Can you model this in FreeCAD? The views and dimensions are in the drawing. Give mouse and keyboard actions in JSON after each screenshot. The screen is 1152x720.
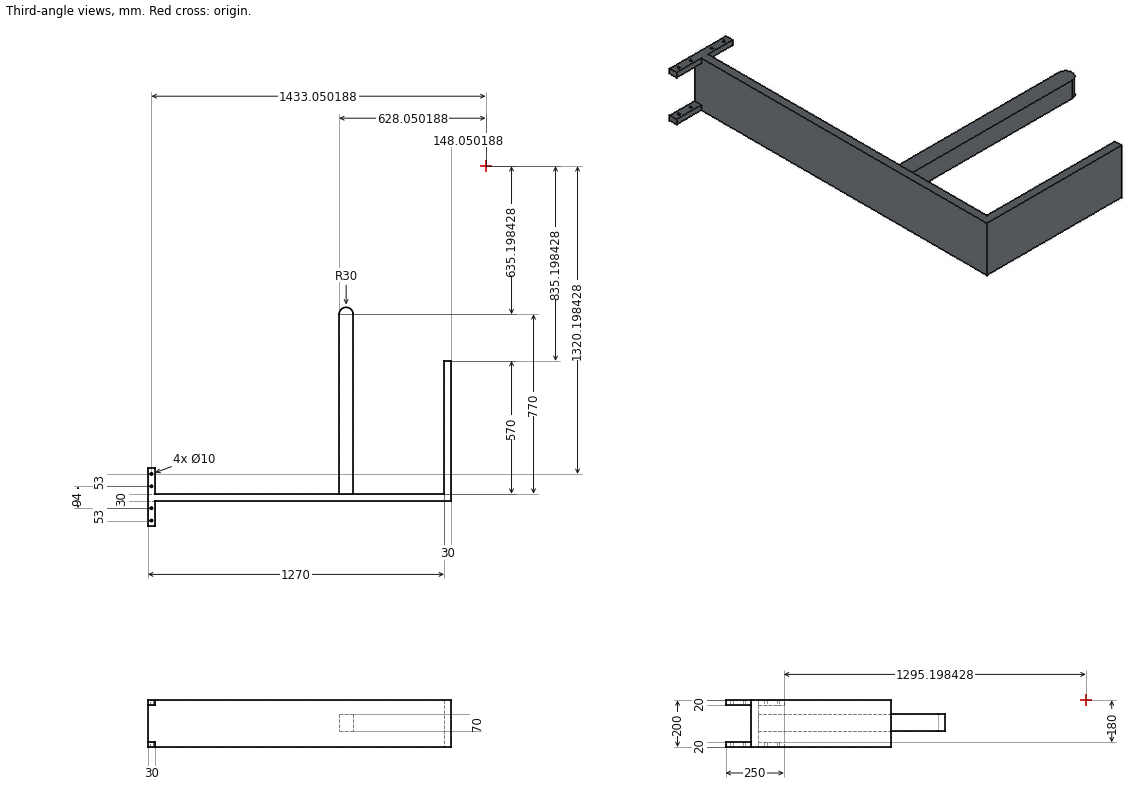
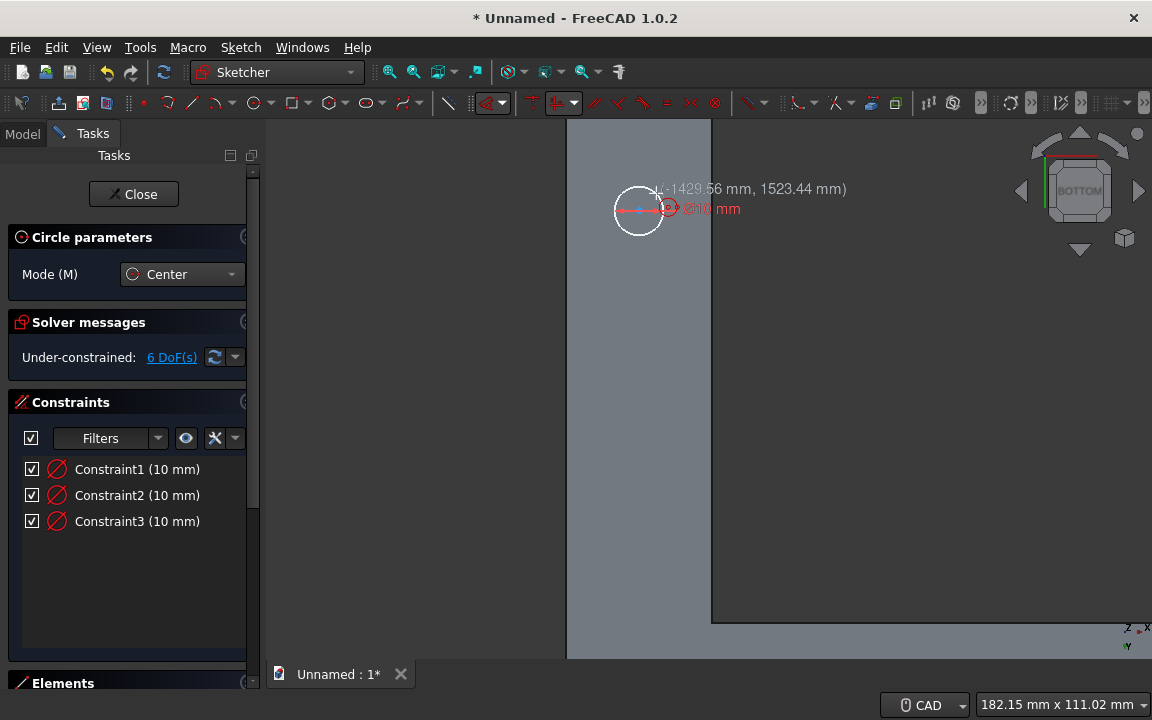
{"action": "left_click", "coordinate": [639, 468]}
{"action": "mouse_move", "coordinate": [656, 450]}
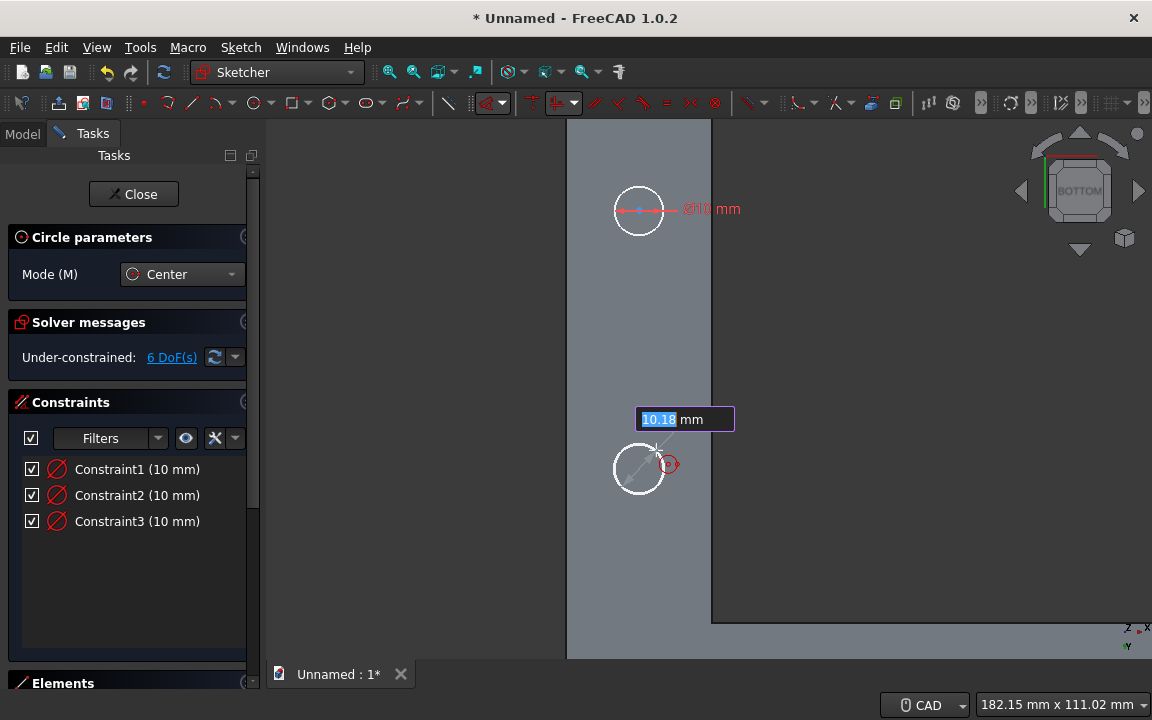
{"action": "type", "text": "10"}
{"action": "key", "text": "Return"}
{"action": "key", "text": "Escape"}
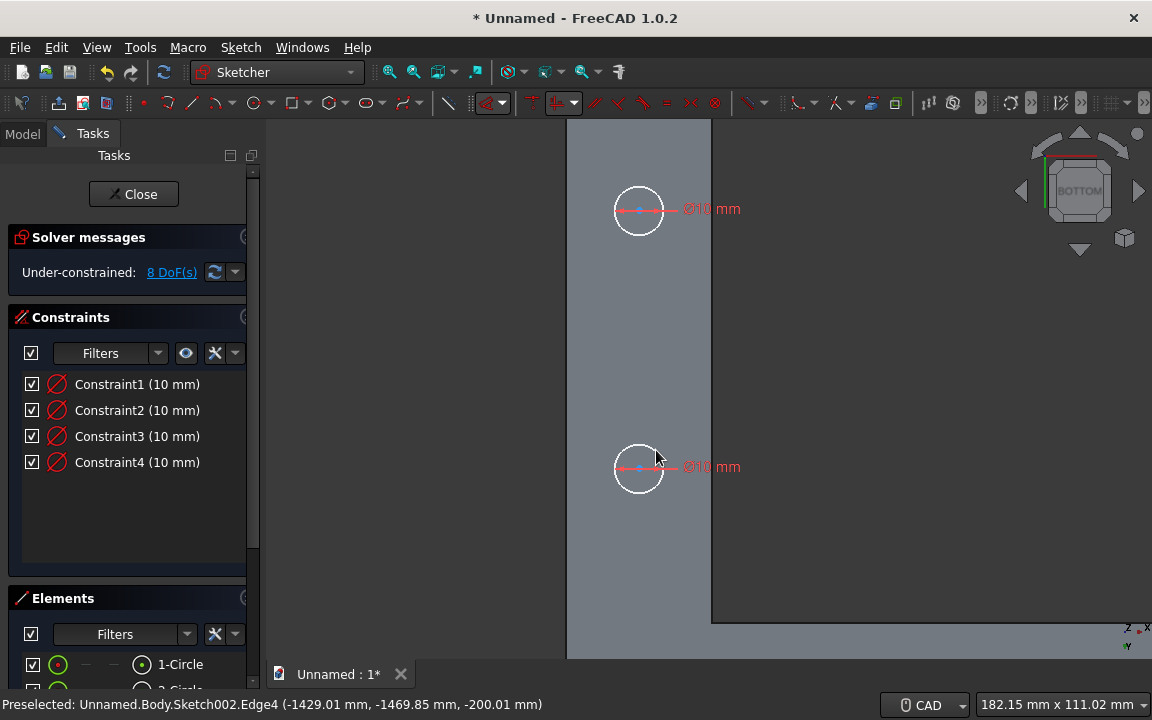
{"action": "scroll", "coordinate": [641, 210], "scroll_direction": "down", "scroll_amount": 5}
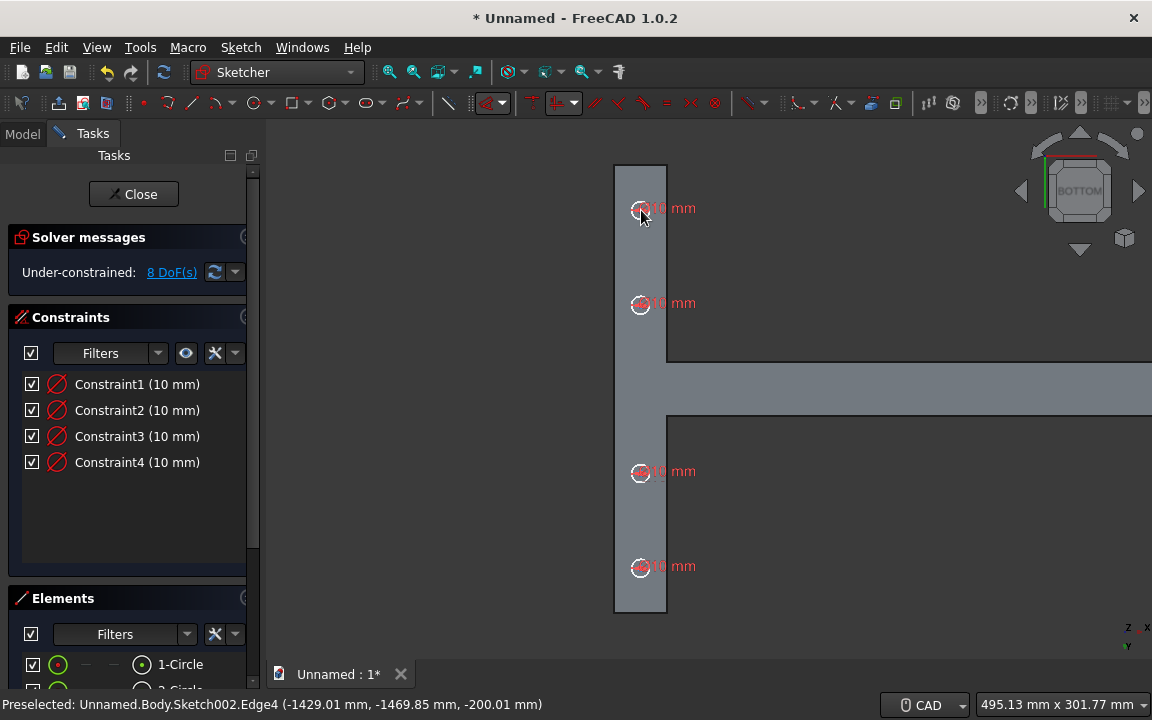
{"action": "left_click", "coordinate": [641, 568]}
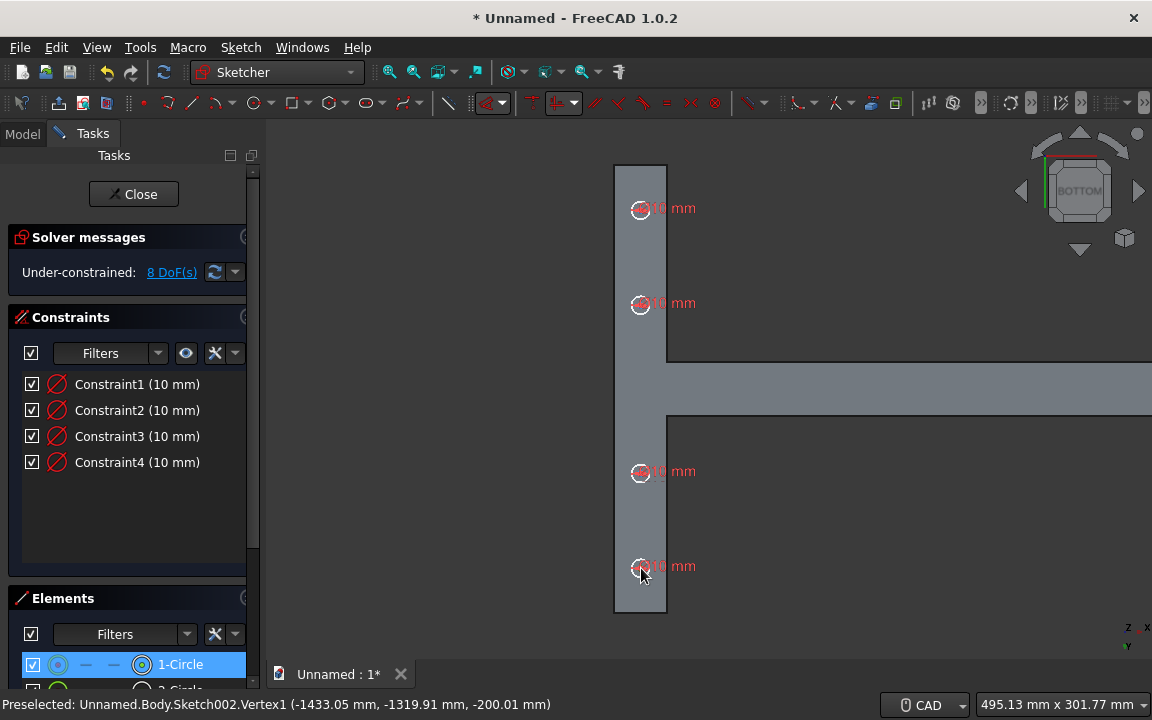
{"action": "left_click", "coordinate": [641, 474]}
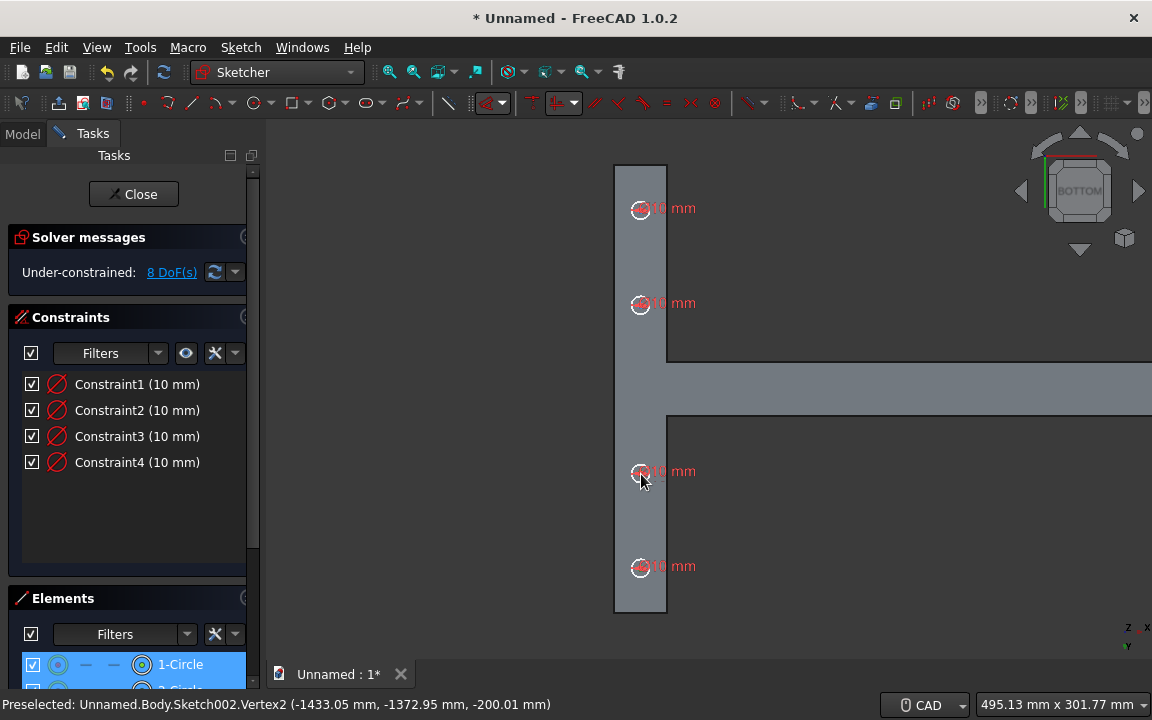
{"action": "left_click", "coordinate": [576, 104]}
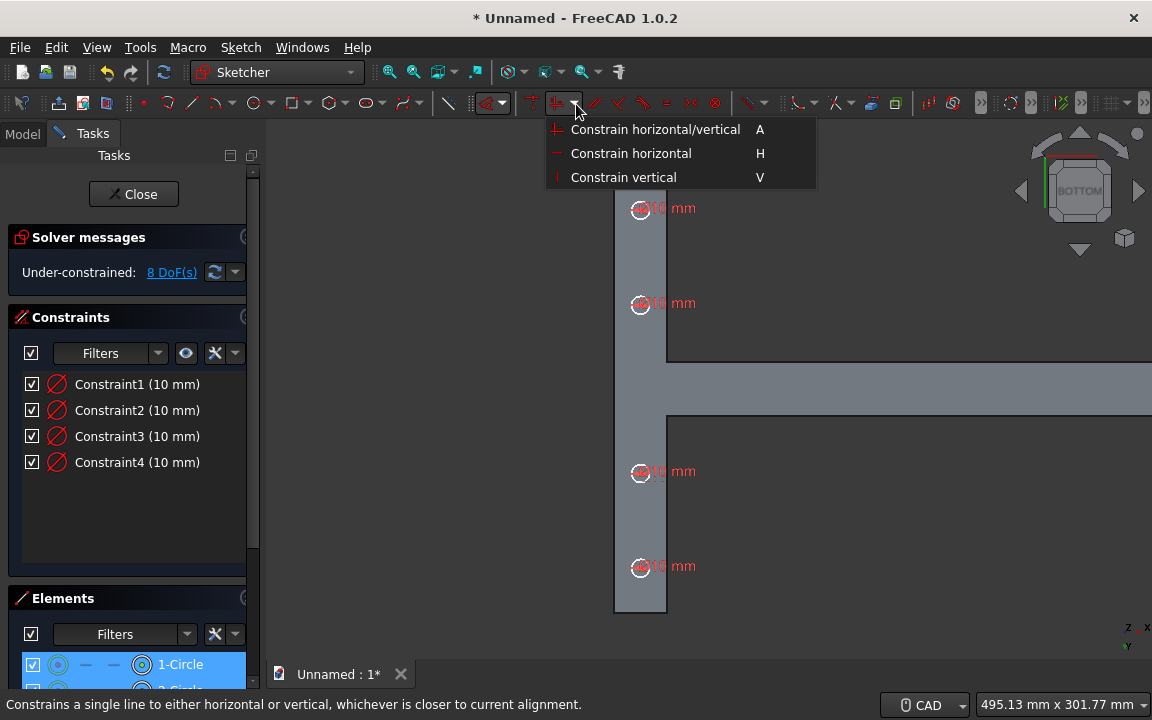
{"action": "left_click", "coordinate": [681, 177]}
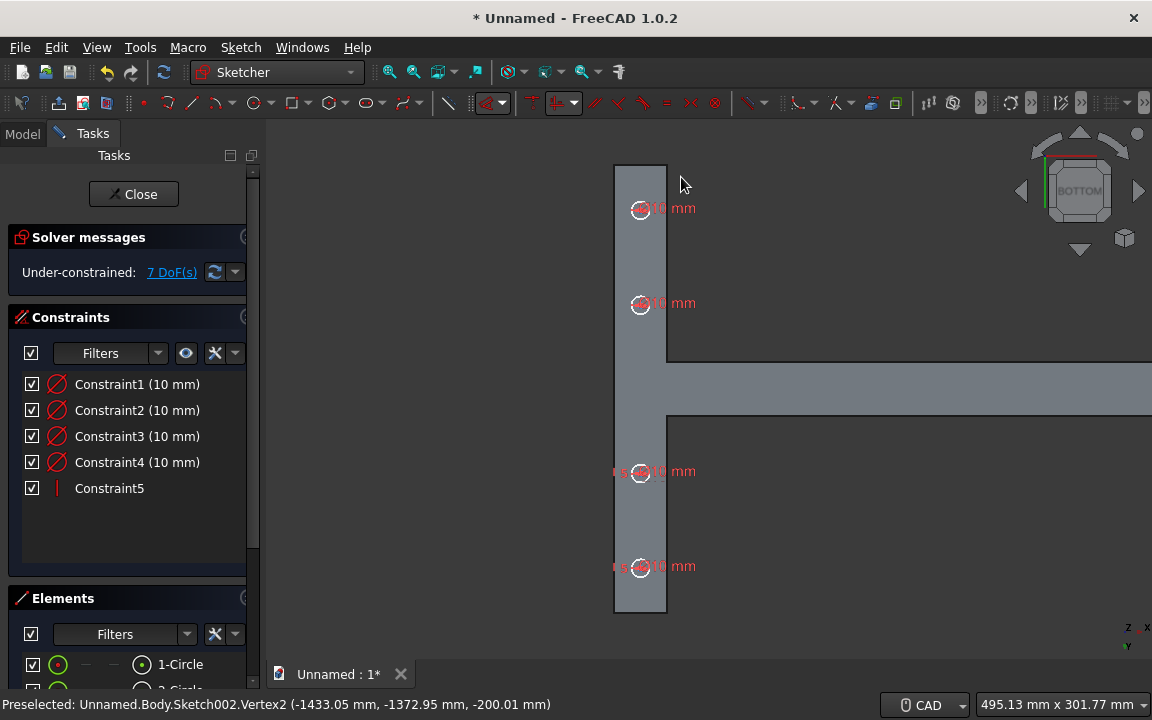
{"action": "left_click", "coordinate": [641, 474]}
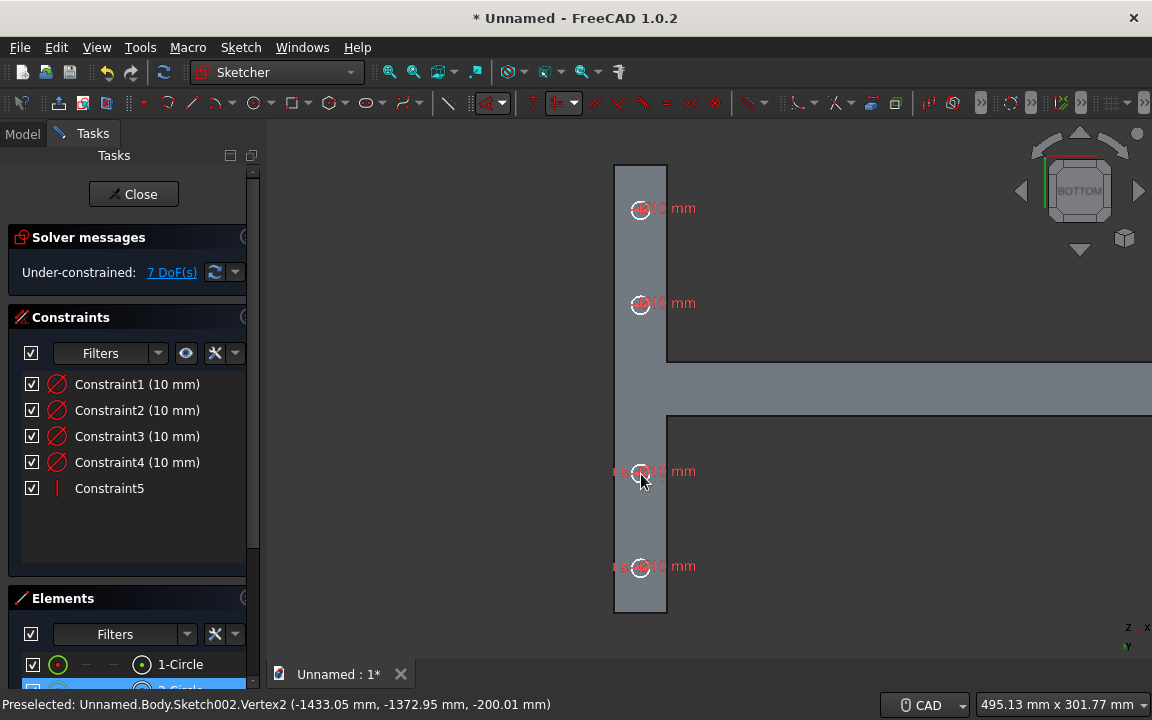
{"action": "left_click", "coordinate": [641, 210]}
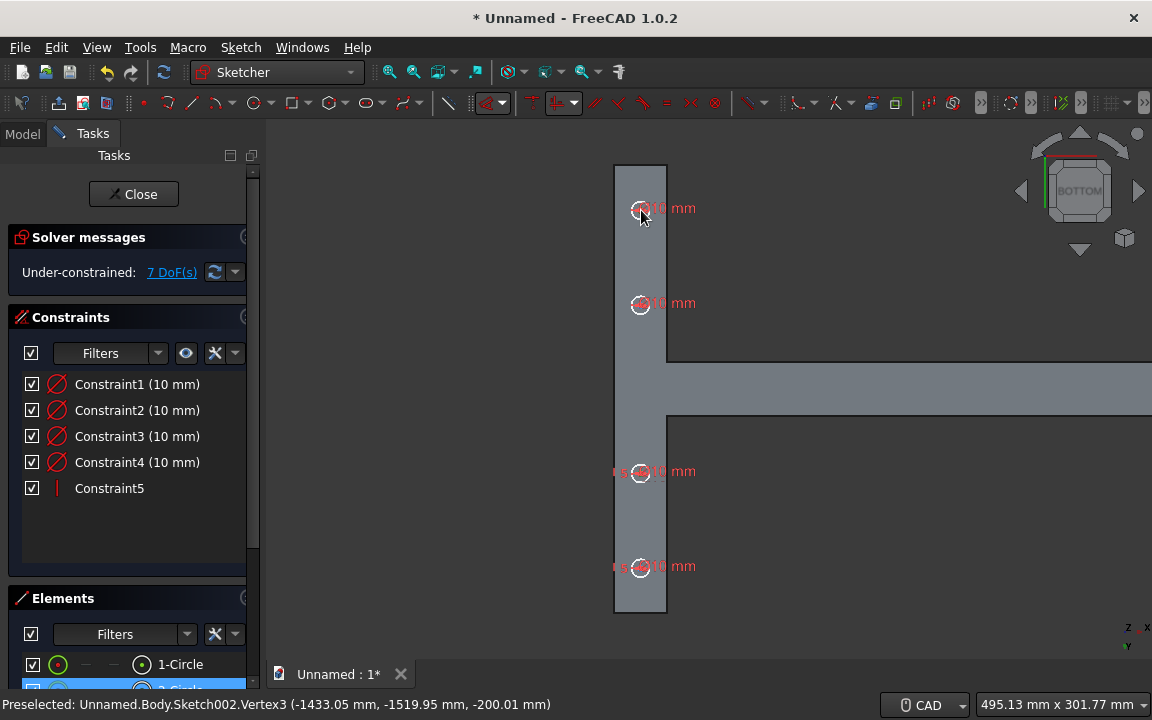
{"action": "key", "text": "v"}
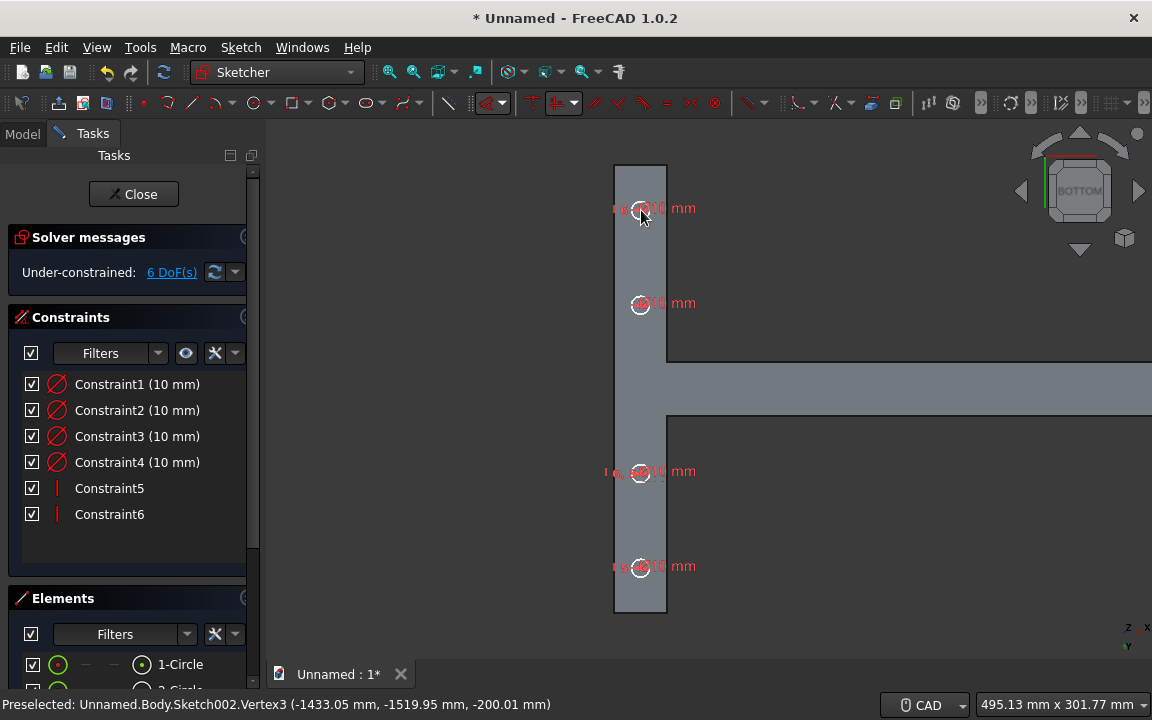
{"action": "left_click", "coordinate": [641, 210]}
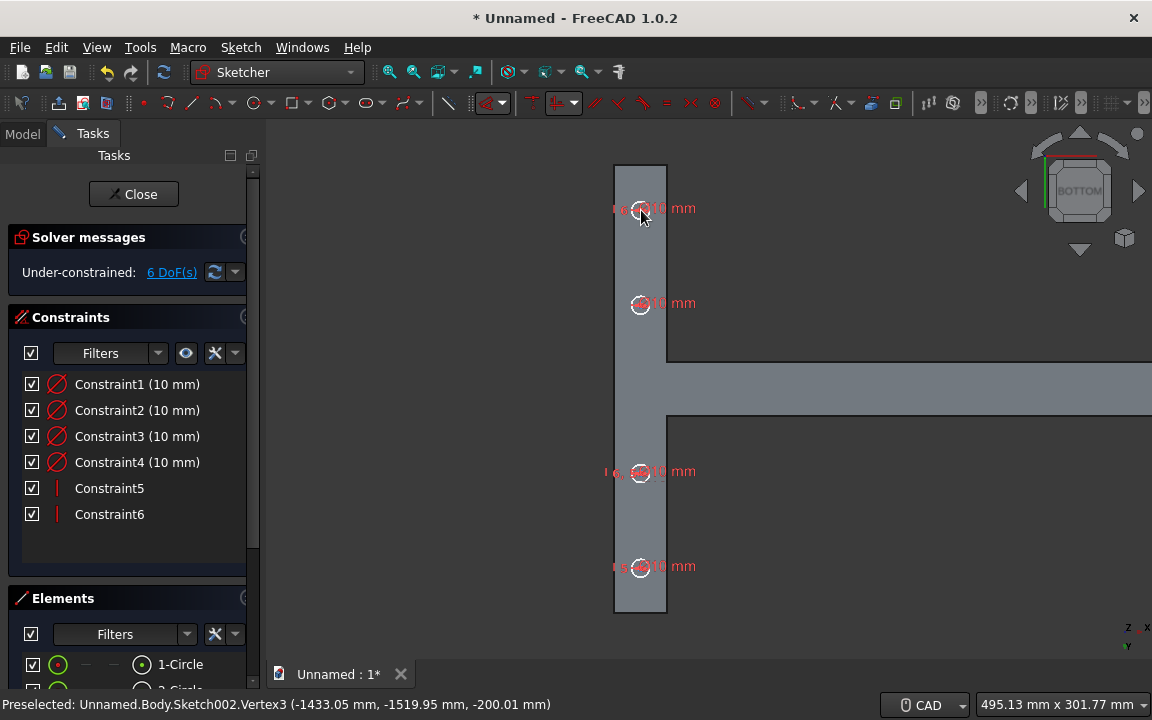
{"action": "left_click", "coordinate": [641, 305]}